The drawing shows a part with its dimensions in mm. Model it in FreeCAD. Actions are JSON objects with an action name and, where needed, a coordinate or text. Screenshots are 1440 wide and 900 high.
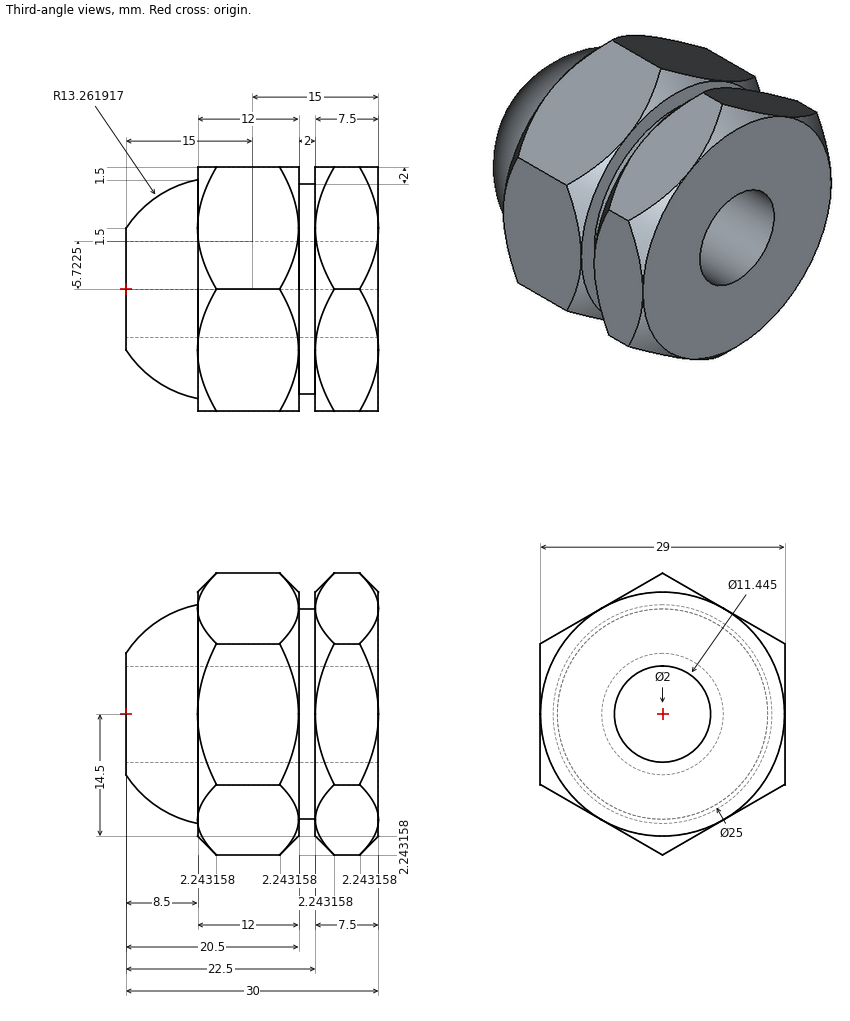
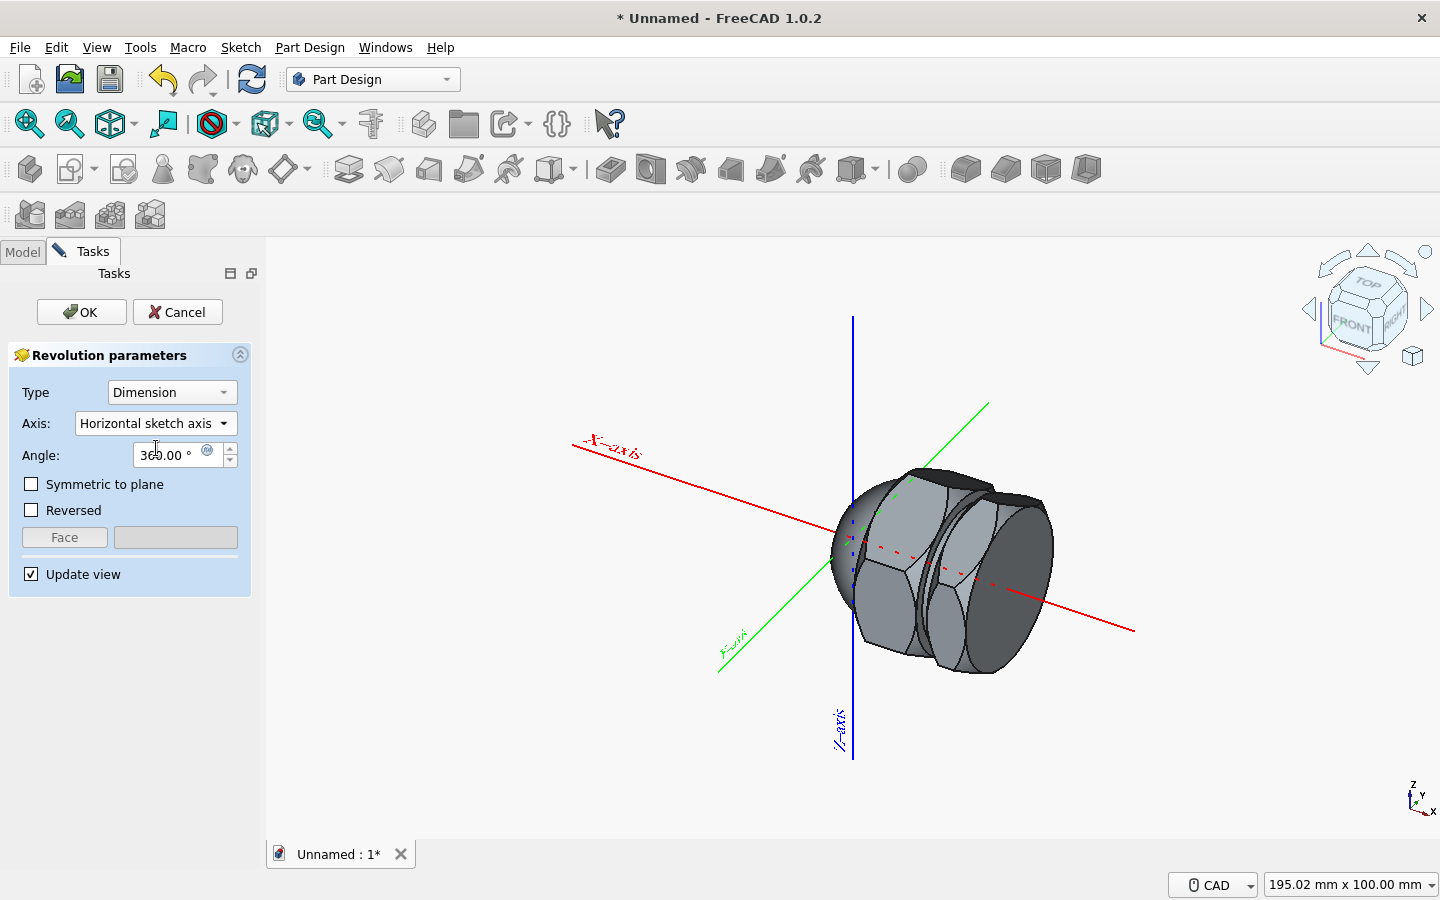
{"action": "left_click", "coordinate": [82, 312]}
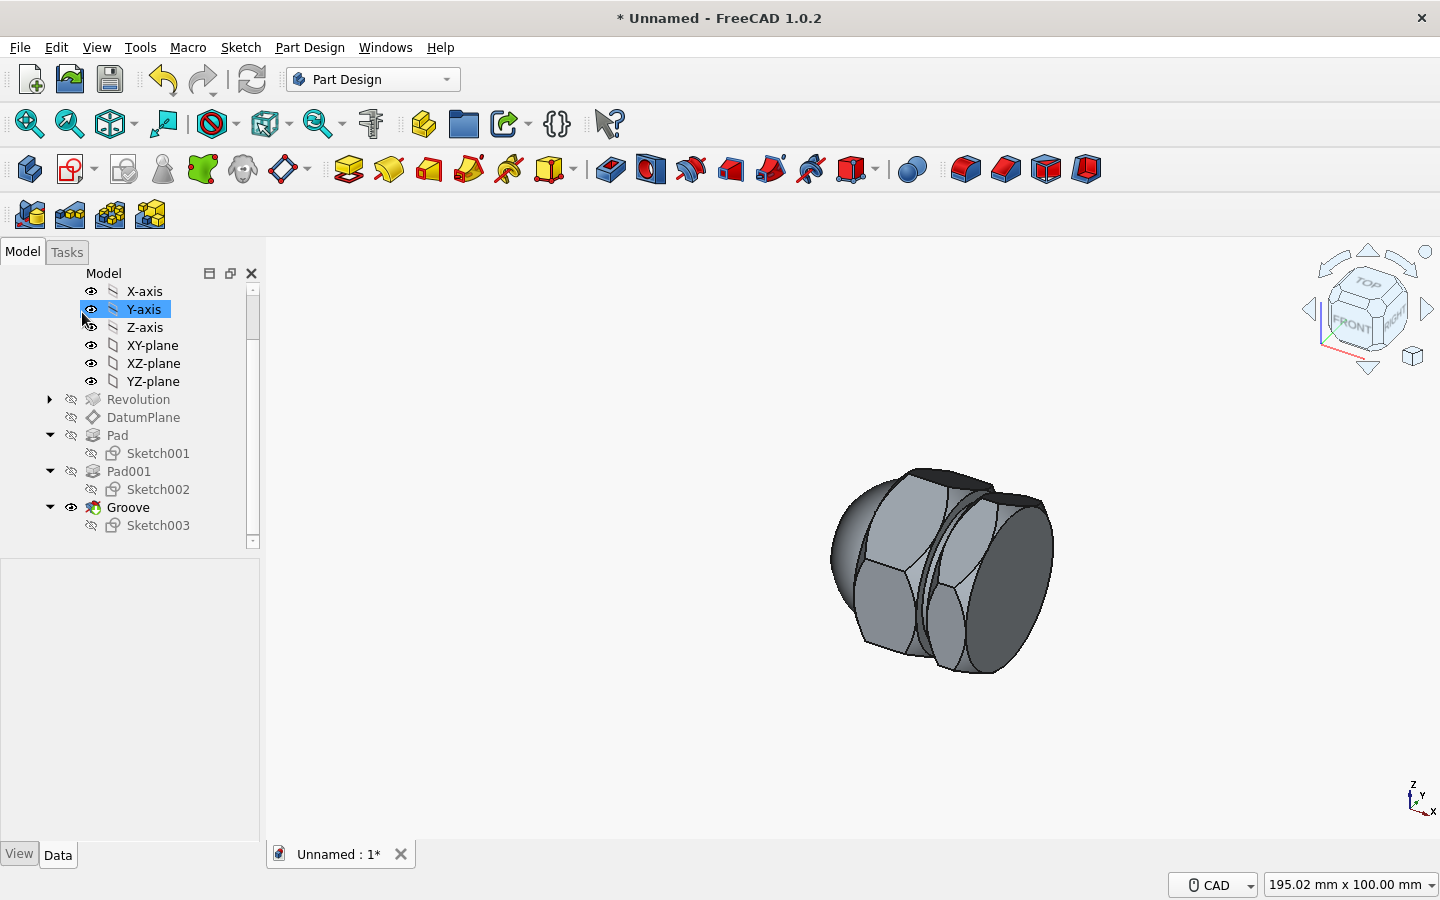
{"action": "key", "text": "6"}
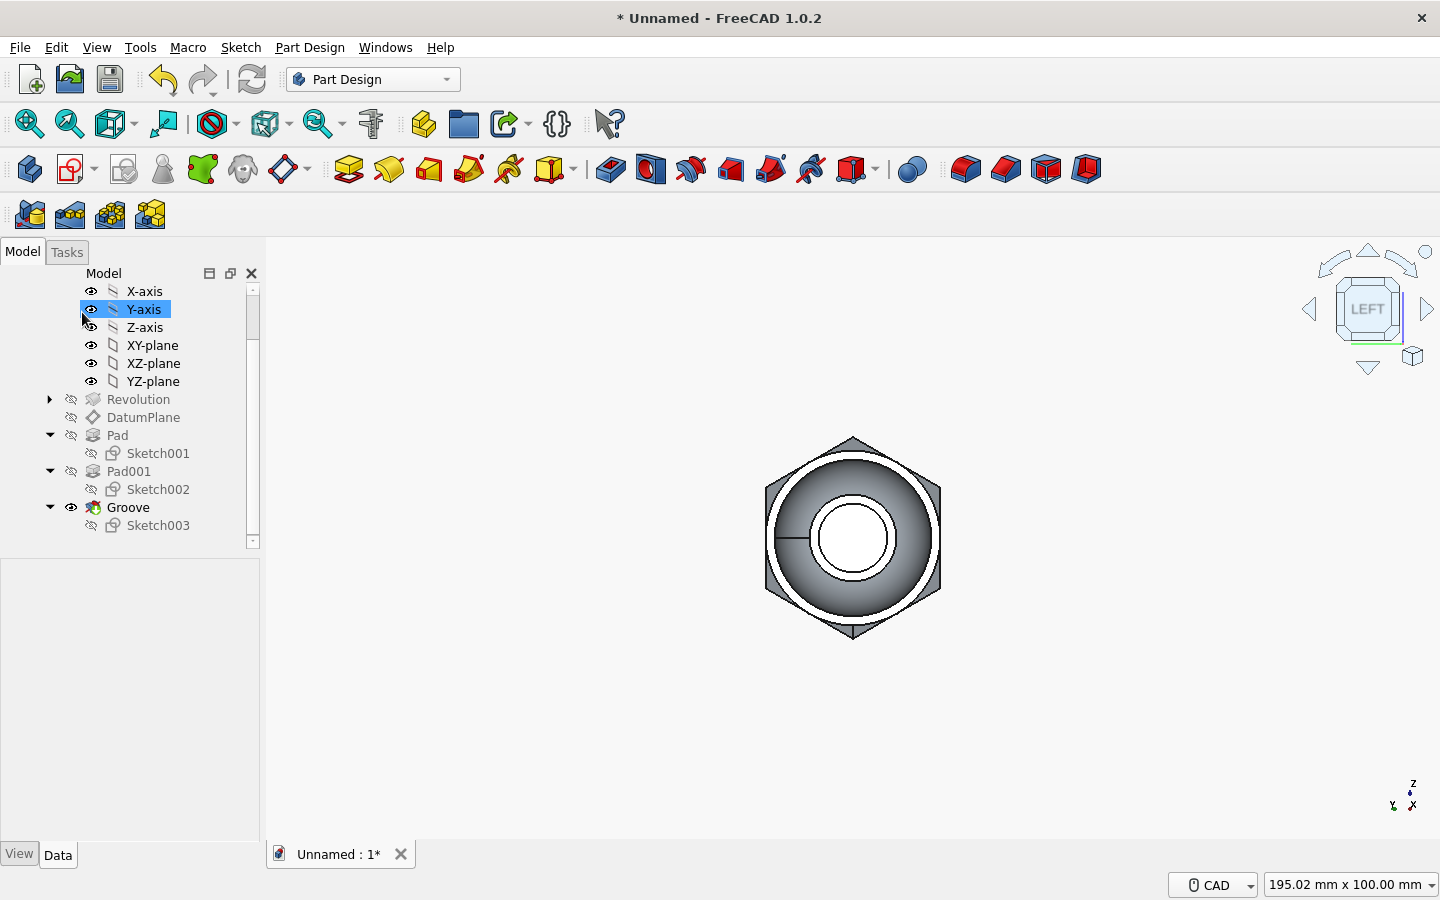
{"action": "left_click", "coordinate": [30, 124]}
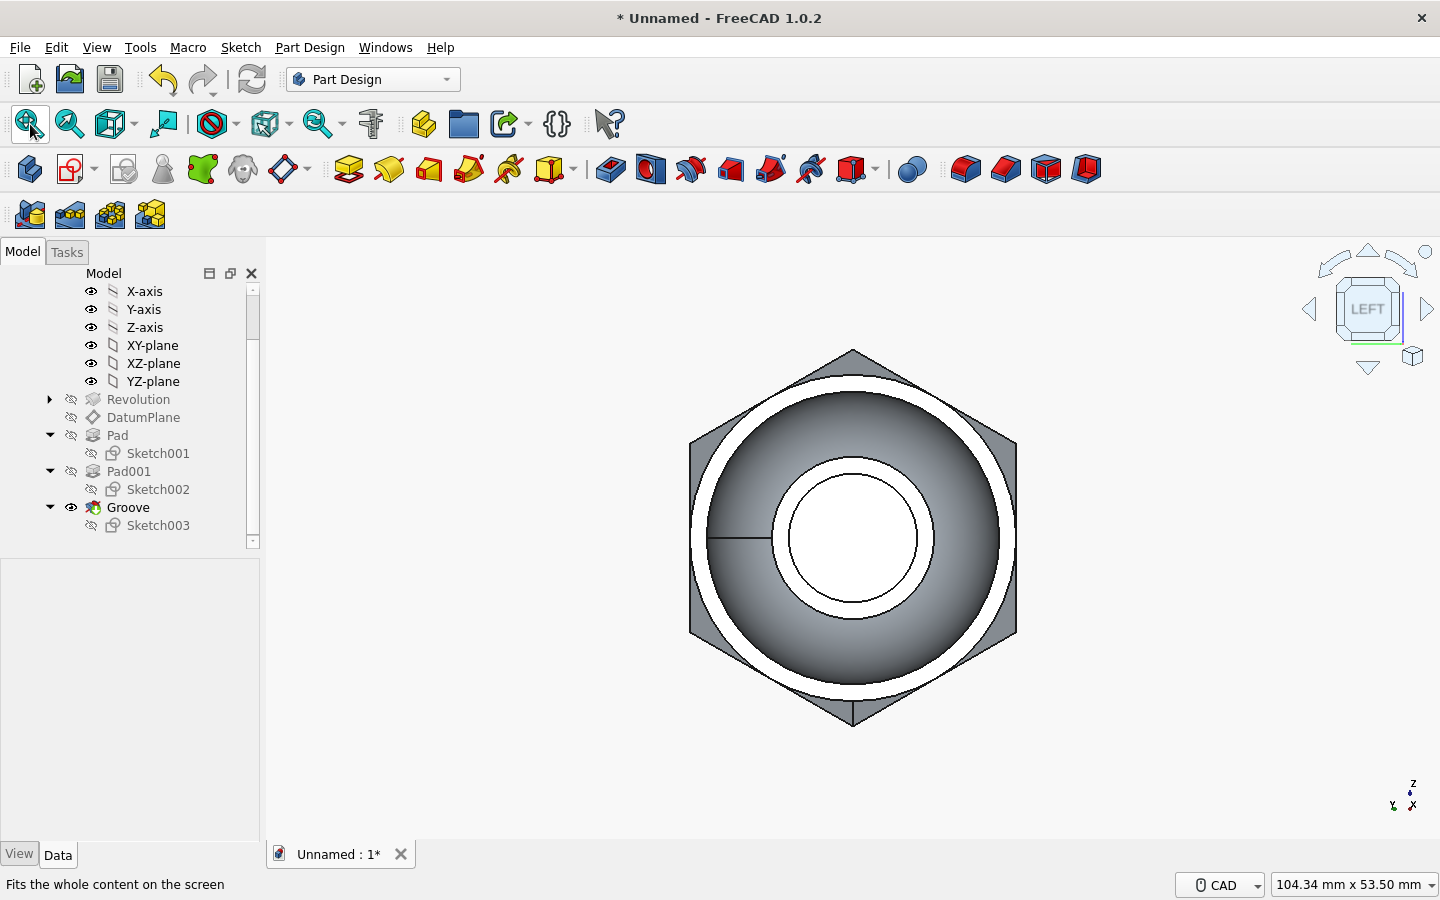
{"action": "left_click", "coordinate": [853, 537]}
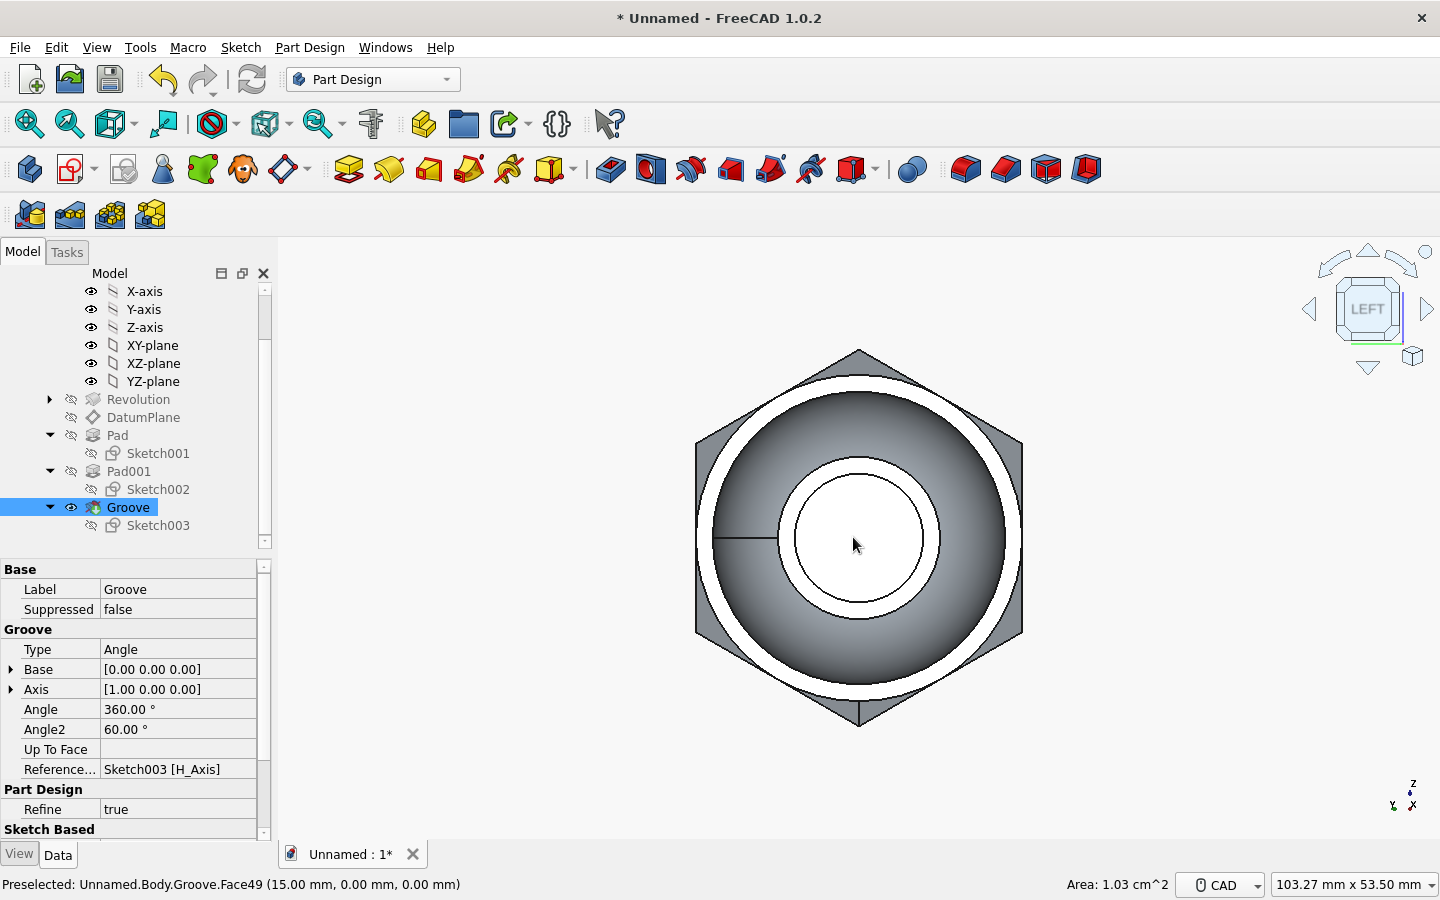
{"action": "left_click", "coordinate": [70, 170]}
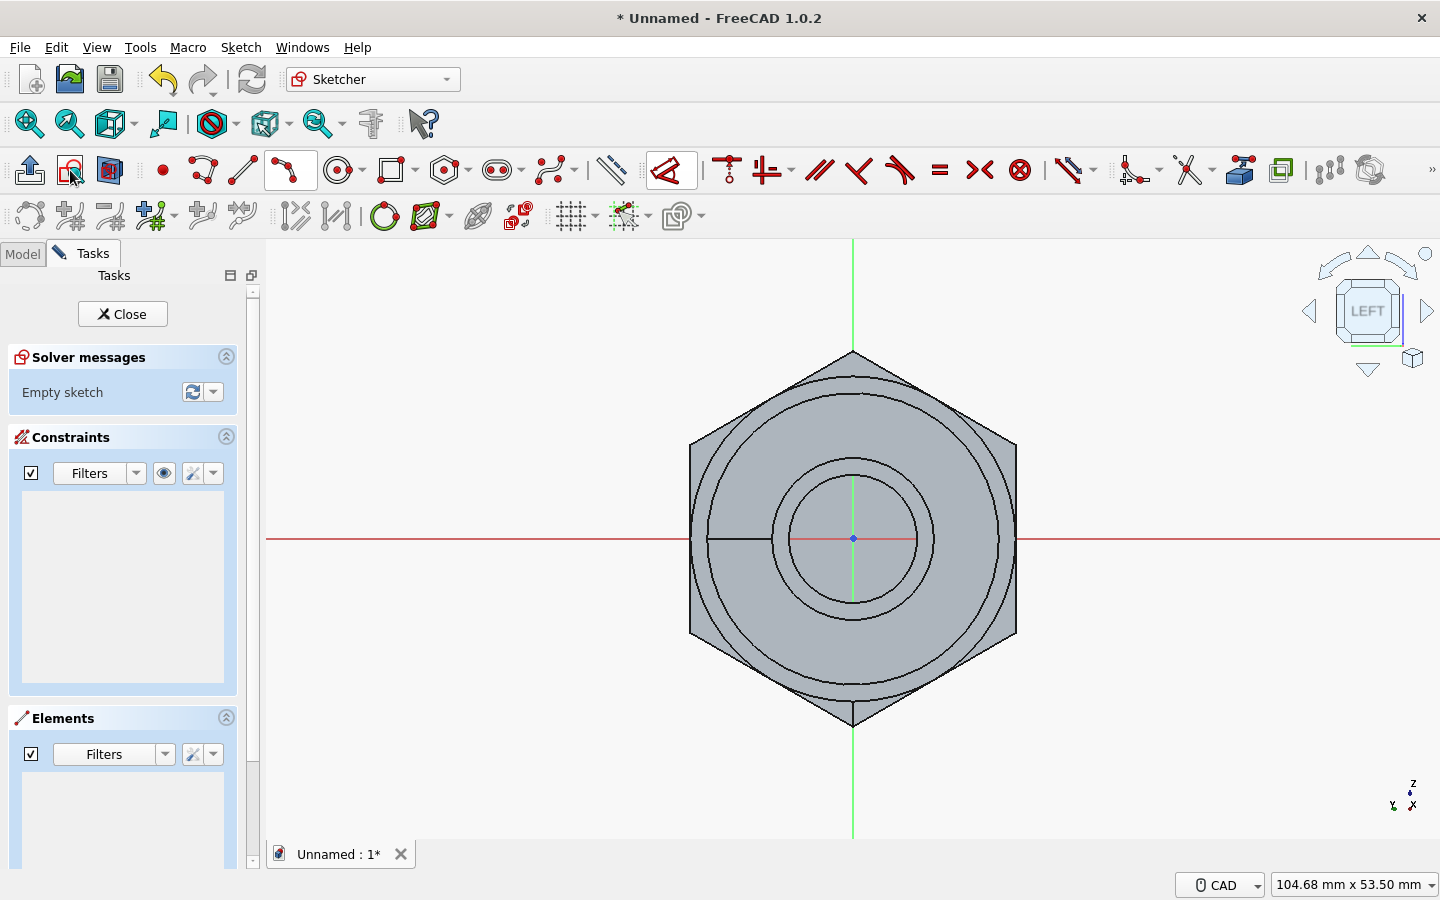
{"action": "left_click", "coordinate": [110, 170]}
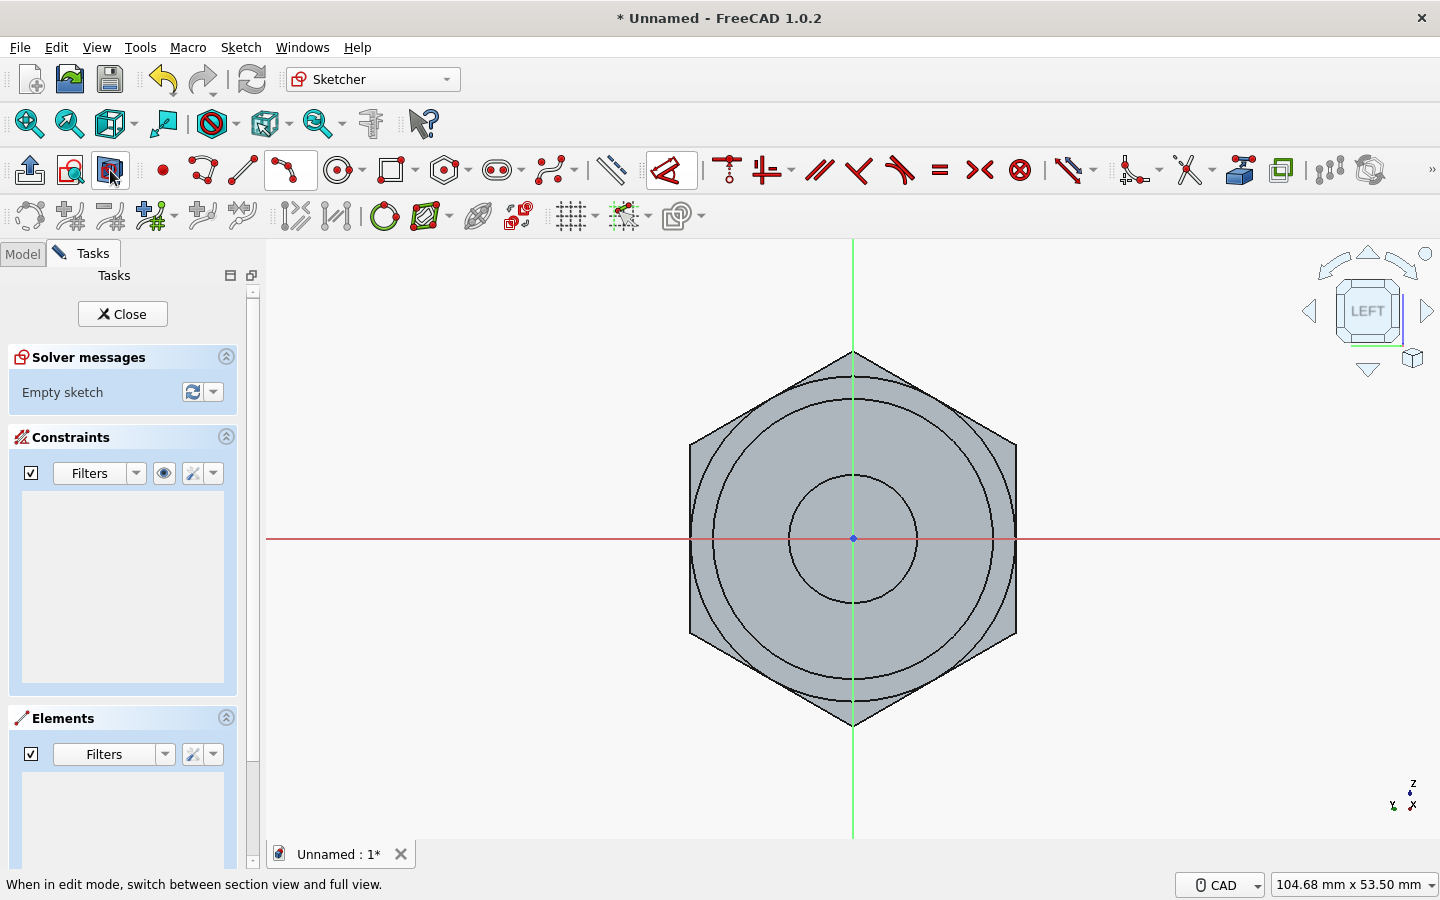
{"action": "scroll", "coordinate": [857, 539], "scroll_direction": "up", "scroll_amount": 14}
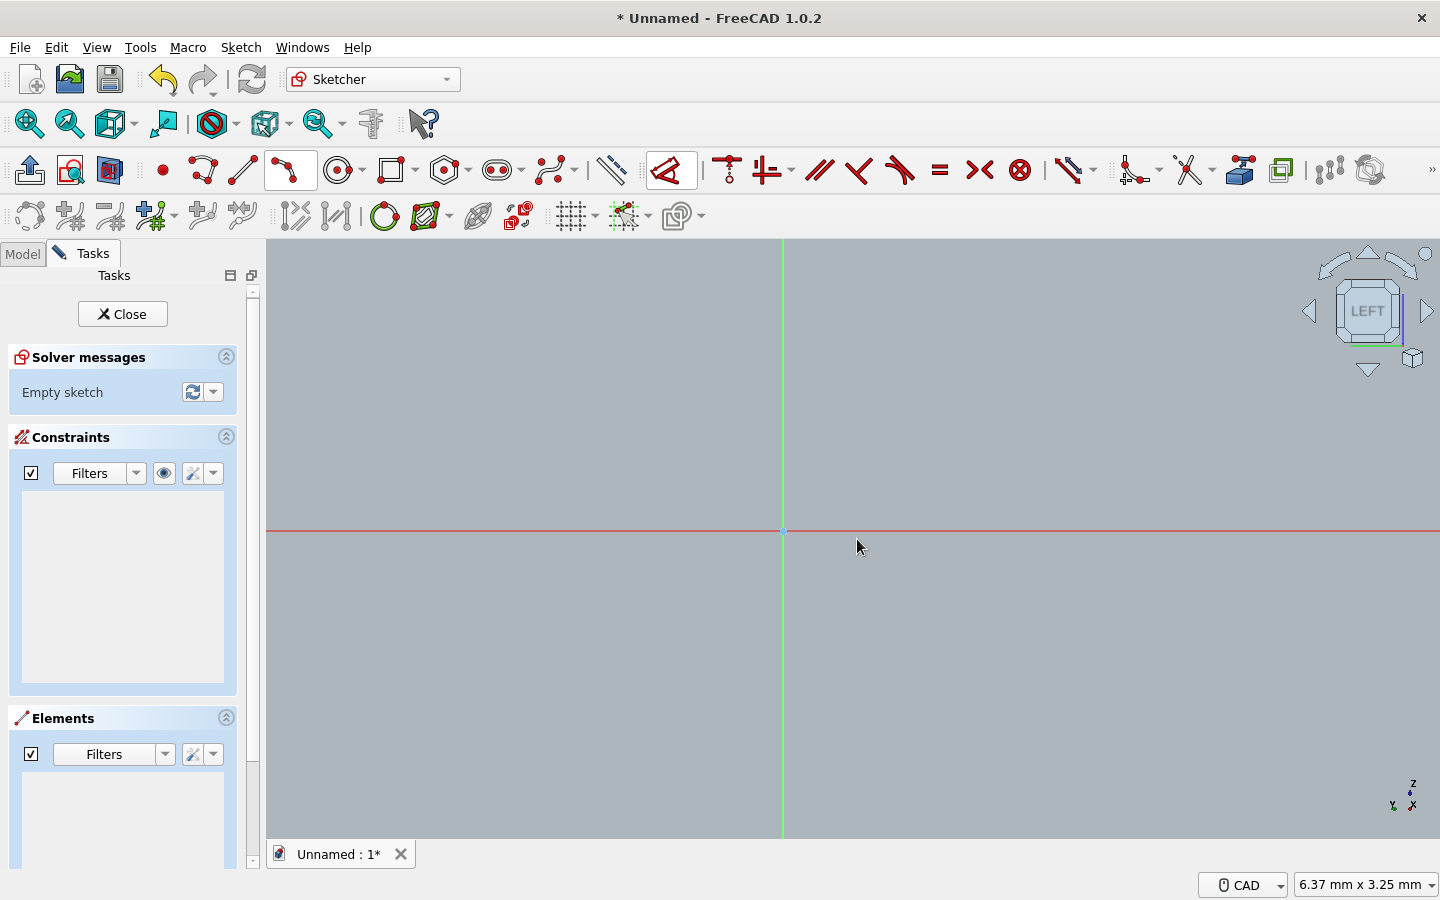
{"action": "left_click", "coordinate": [338, 170]}